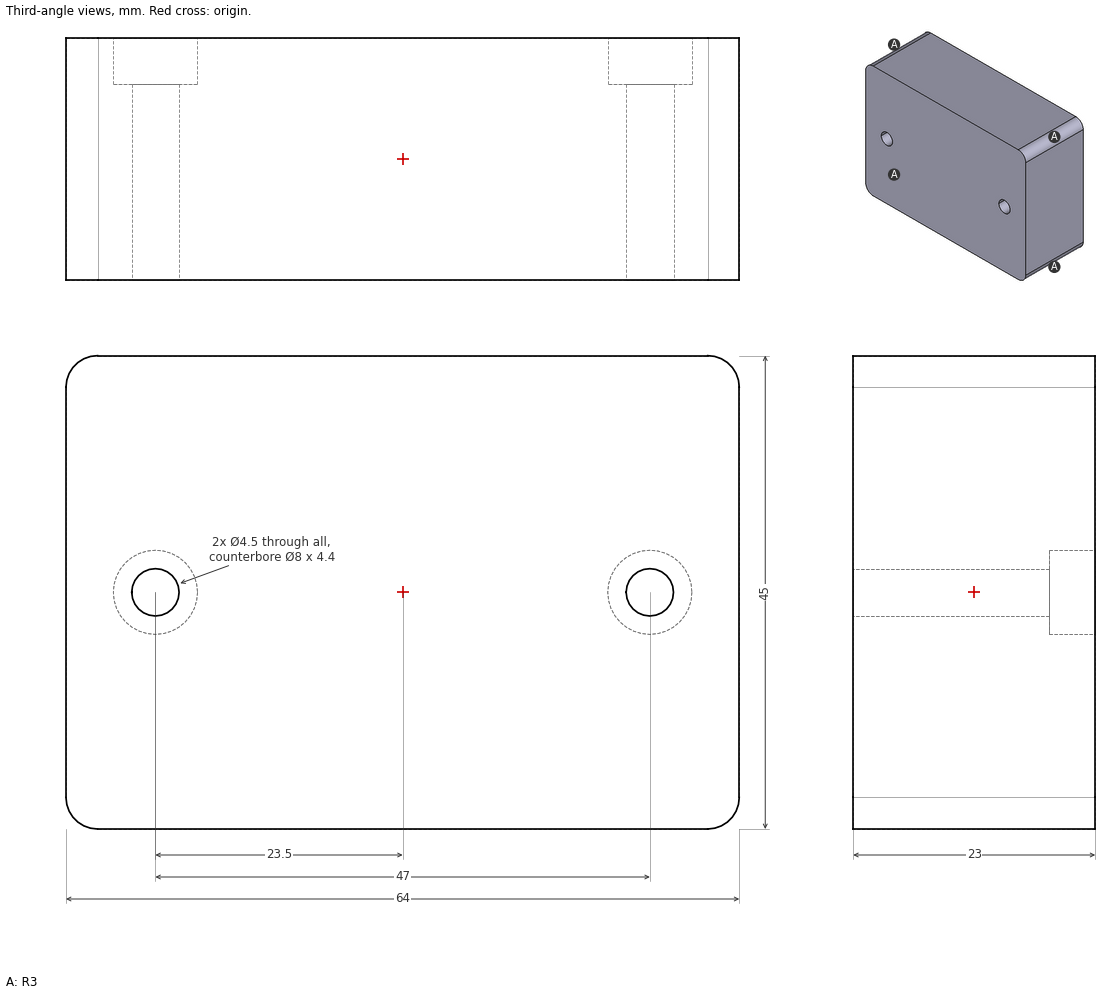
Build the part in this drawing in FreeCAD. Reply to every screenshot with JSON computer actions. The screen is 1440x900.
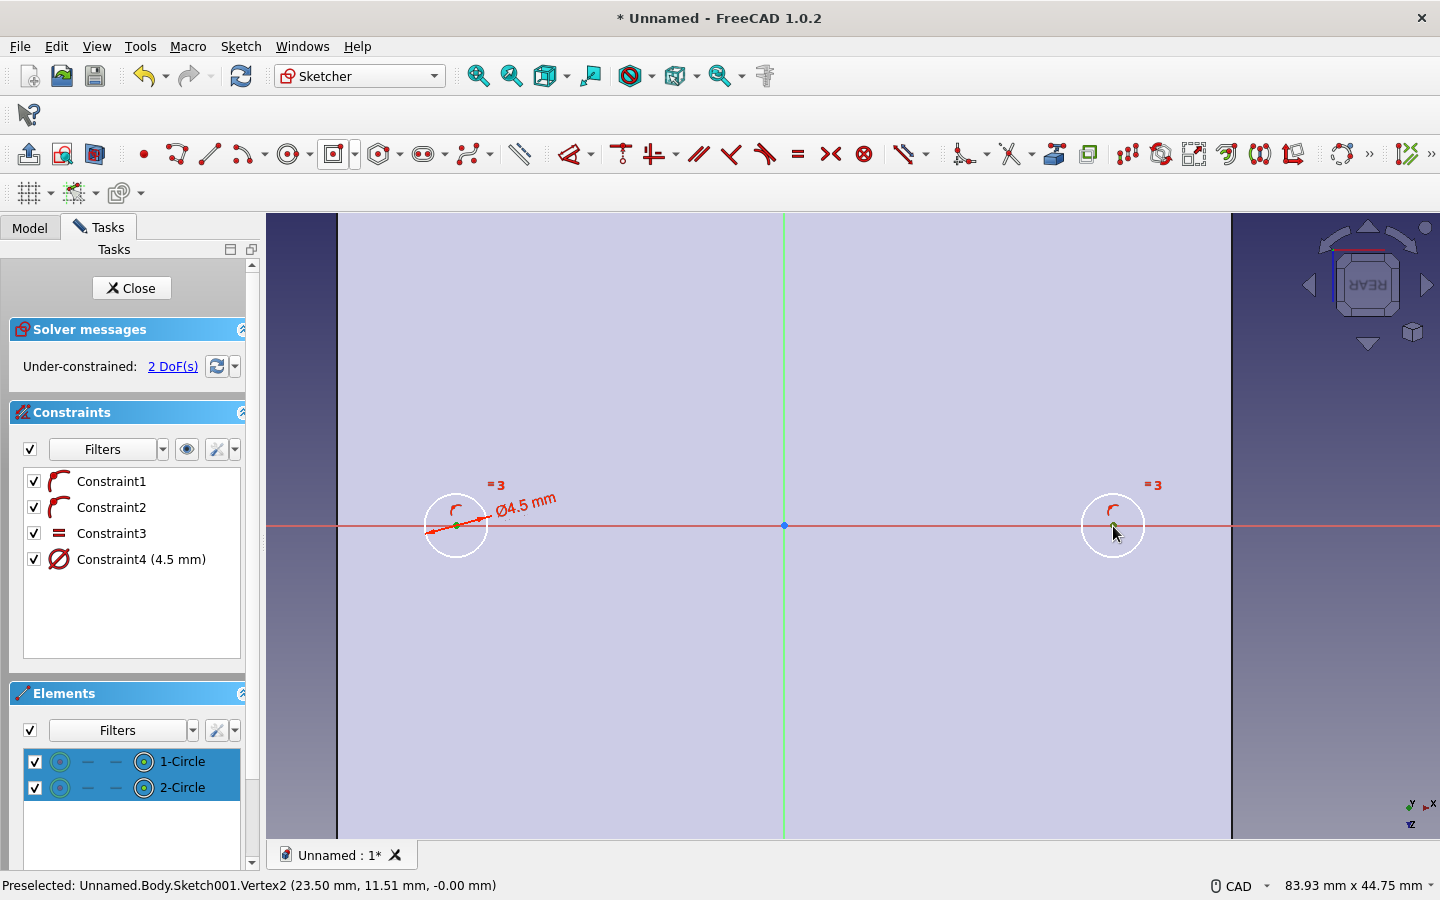
{"action": "left_click", "coordinate": [590, 154]}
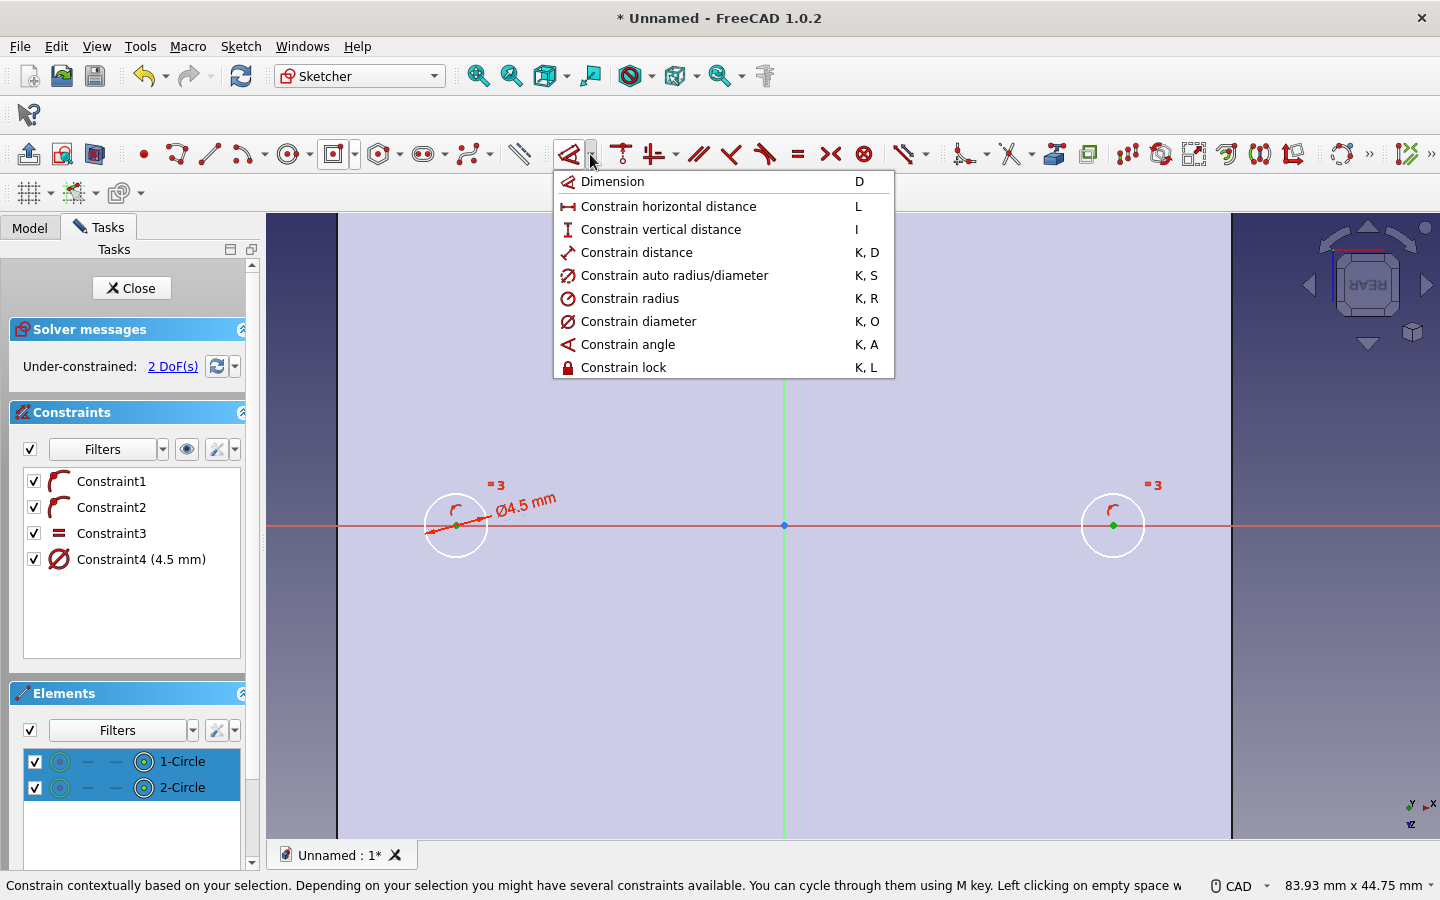
{"action": "left_click", "coordinate": [724, 206]}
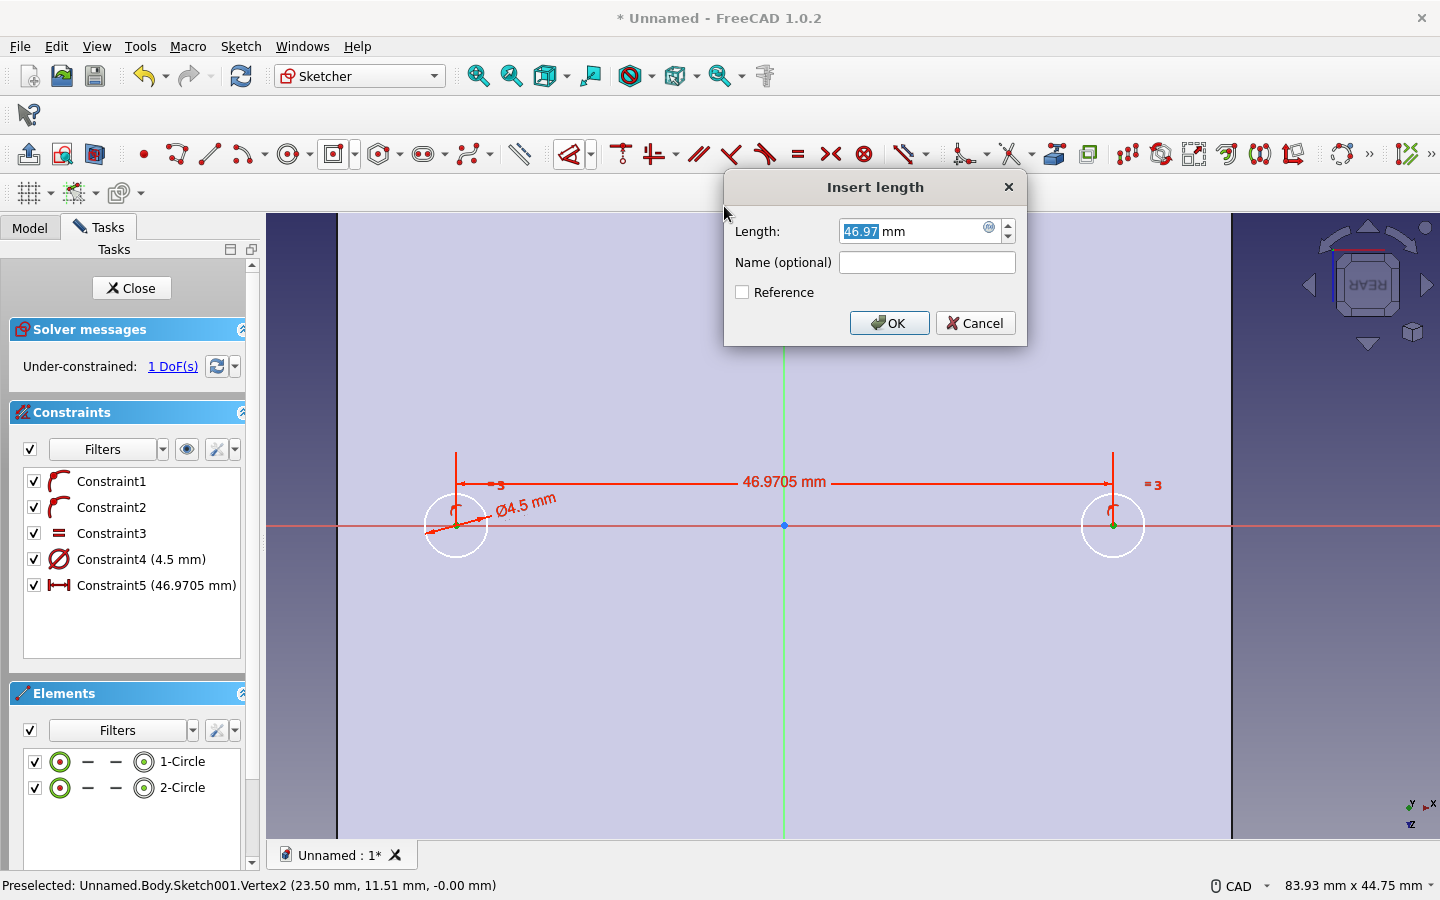
{"action": "type", "text": "47"}
{"action": "key", "text": "Return"}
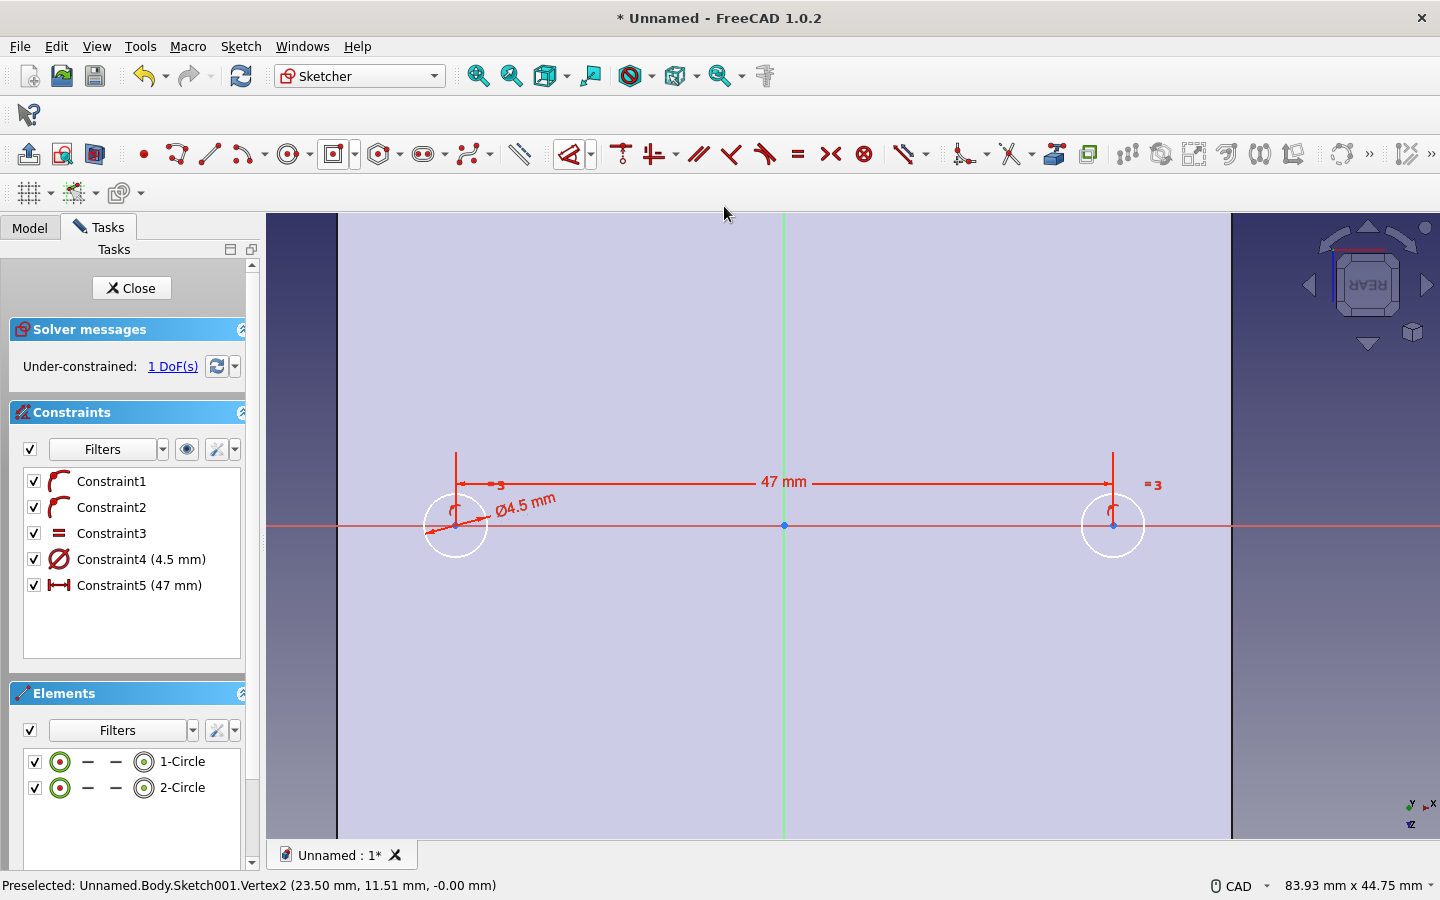
{"action": "left_click", "coordinate": [456, 526]}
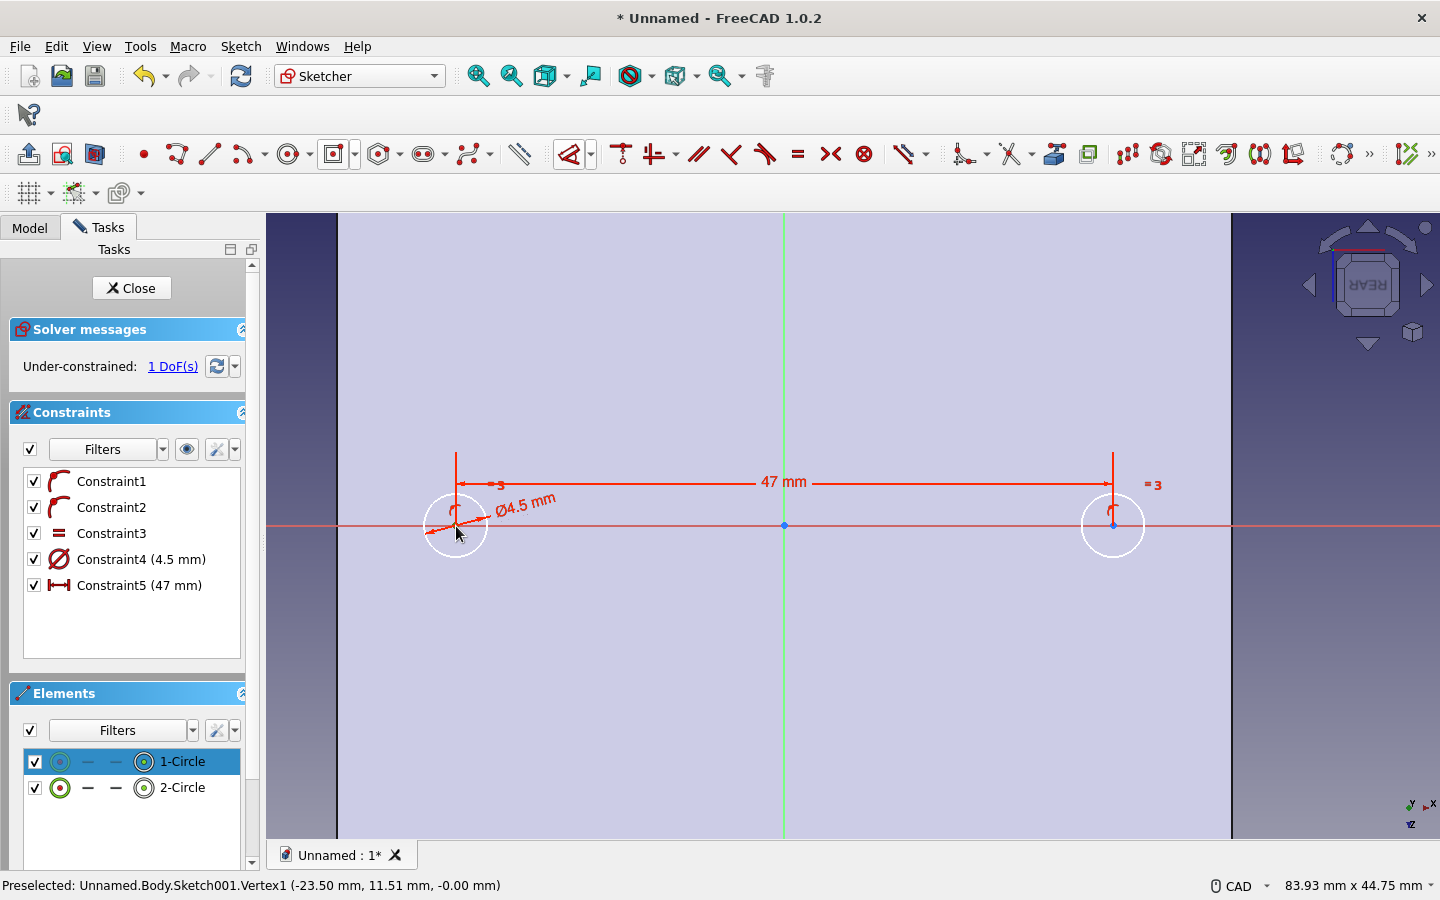
{"action": "key", "text": "l"}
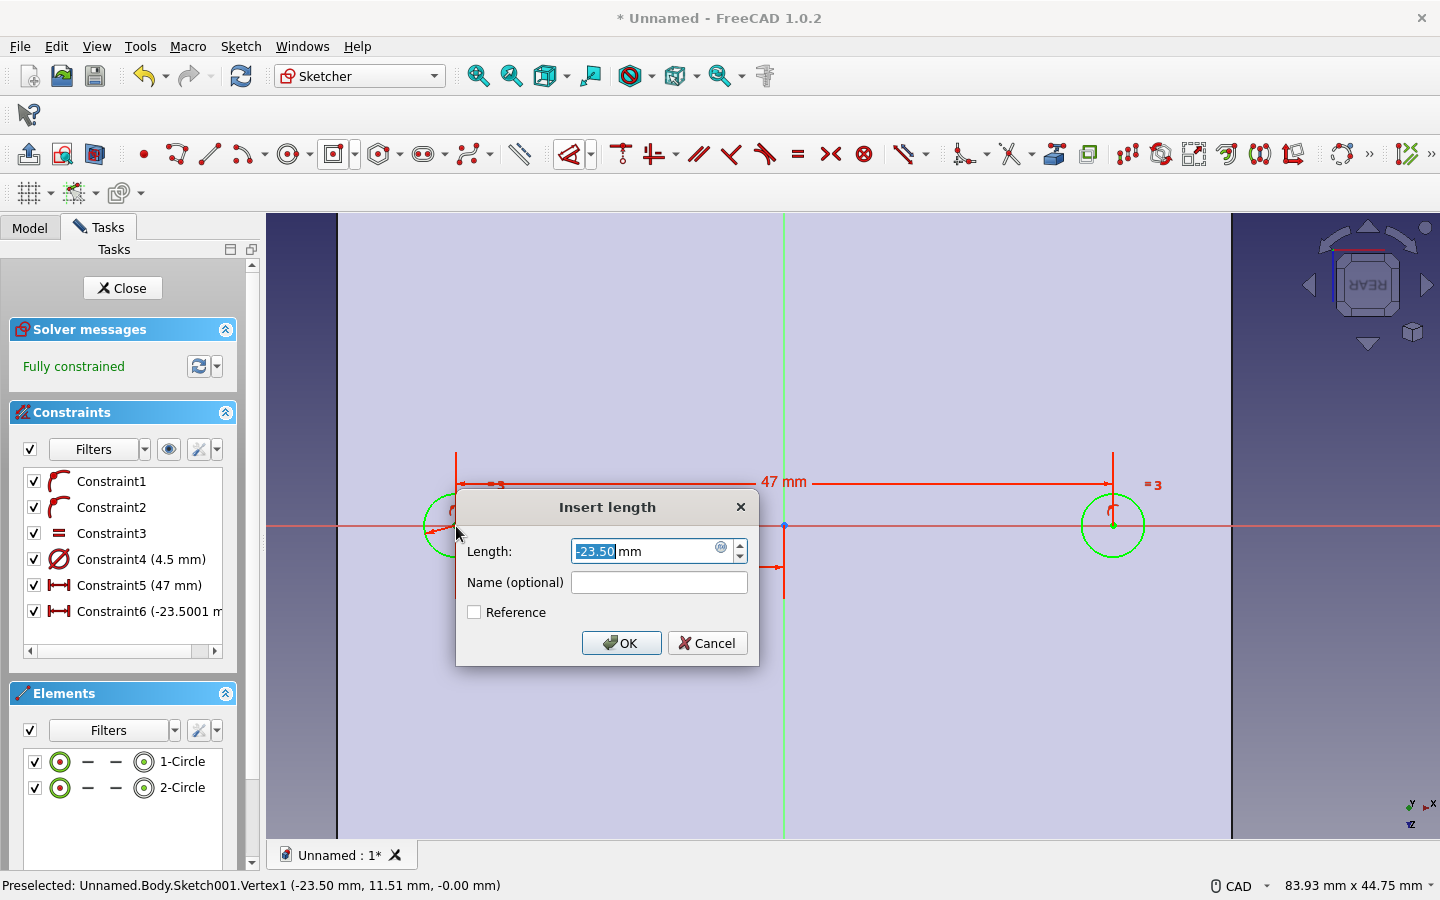
{"action": "type", "text": "-23.5"}
{"action": "key", "text": "Return"}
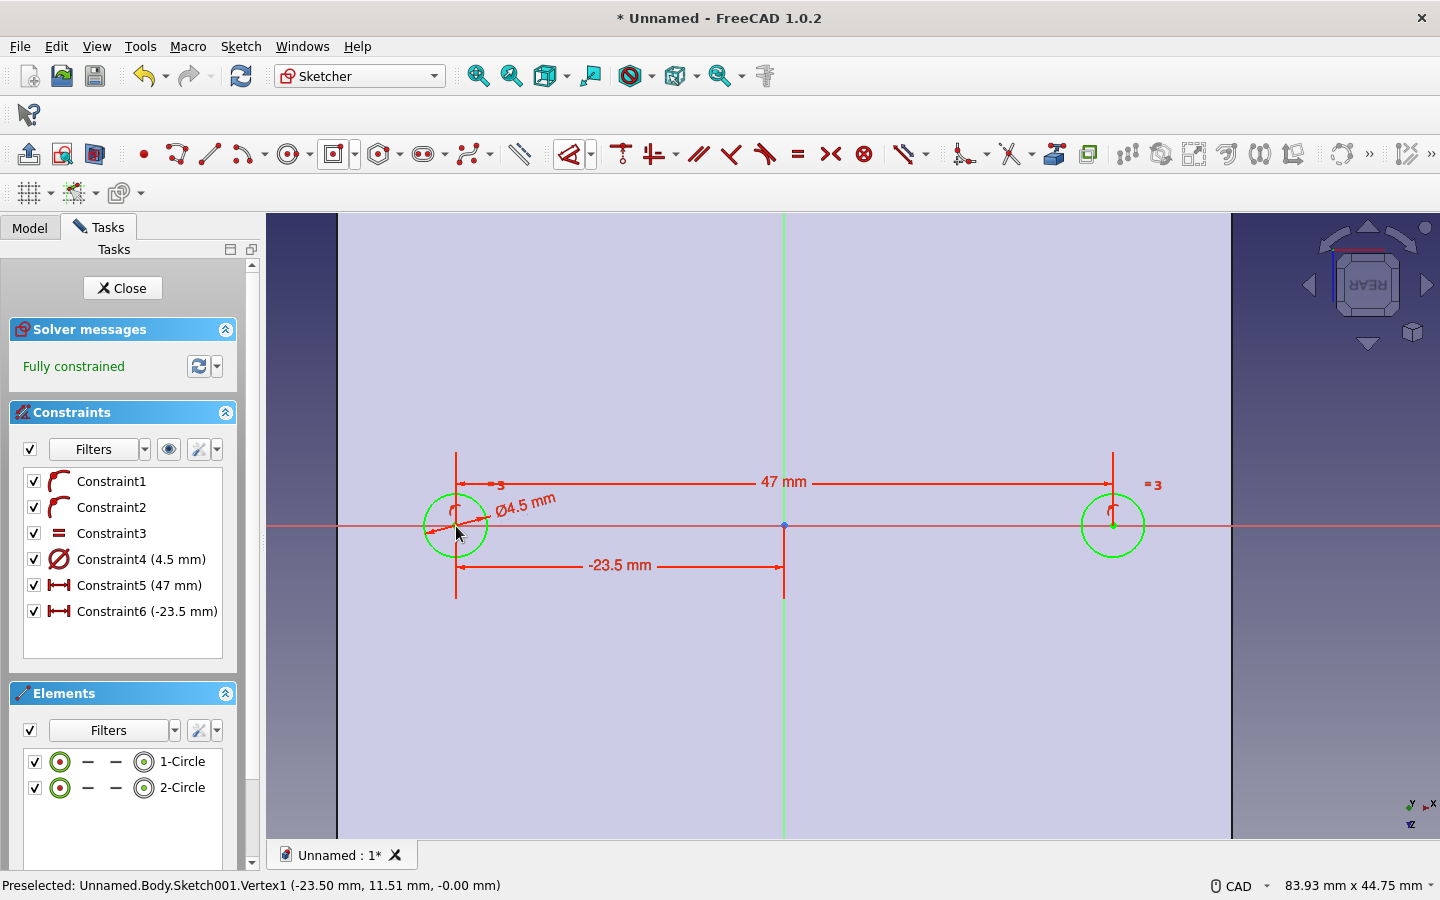
{"action": "left_click", "coordinate": [123, 288]}